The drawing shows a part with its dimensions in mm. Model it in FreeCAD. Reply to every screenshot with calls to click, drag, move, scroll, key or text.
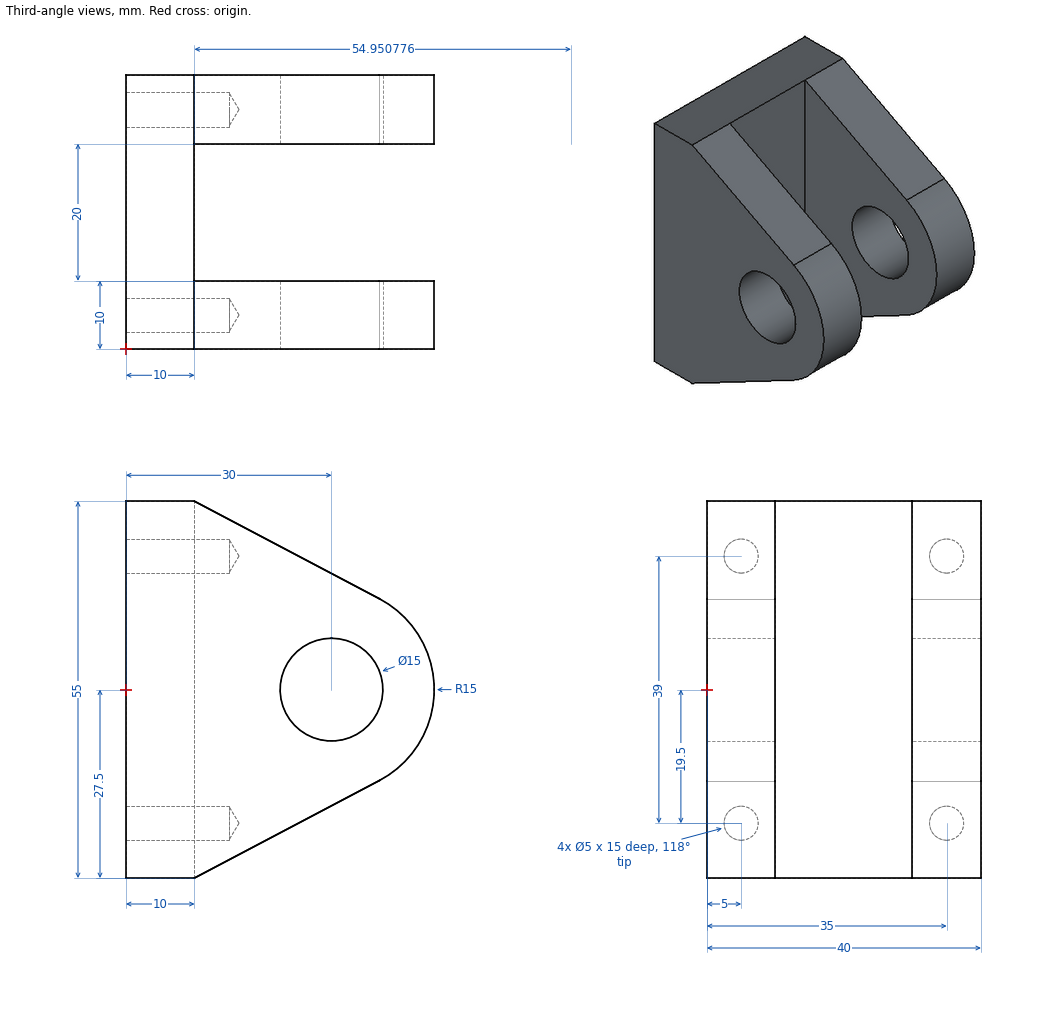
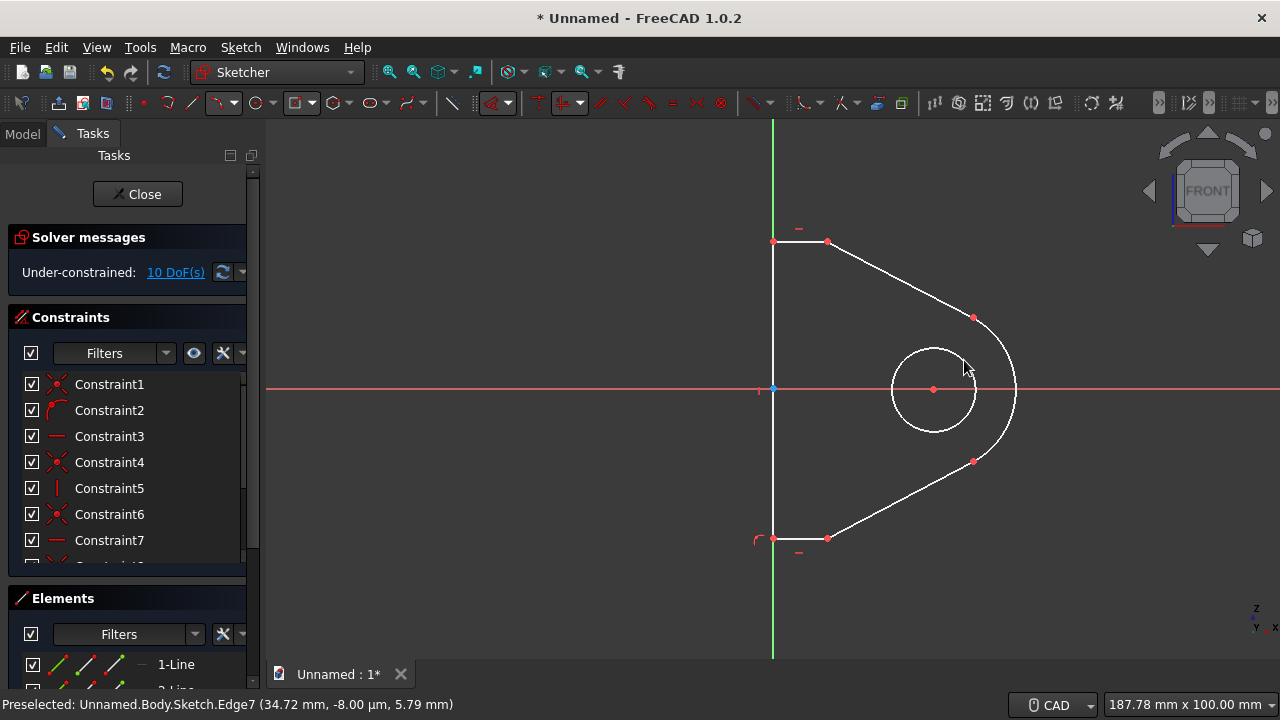
click(929, 485)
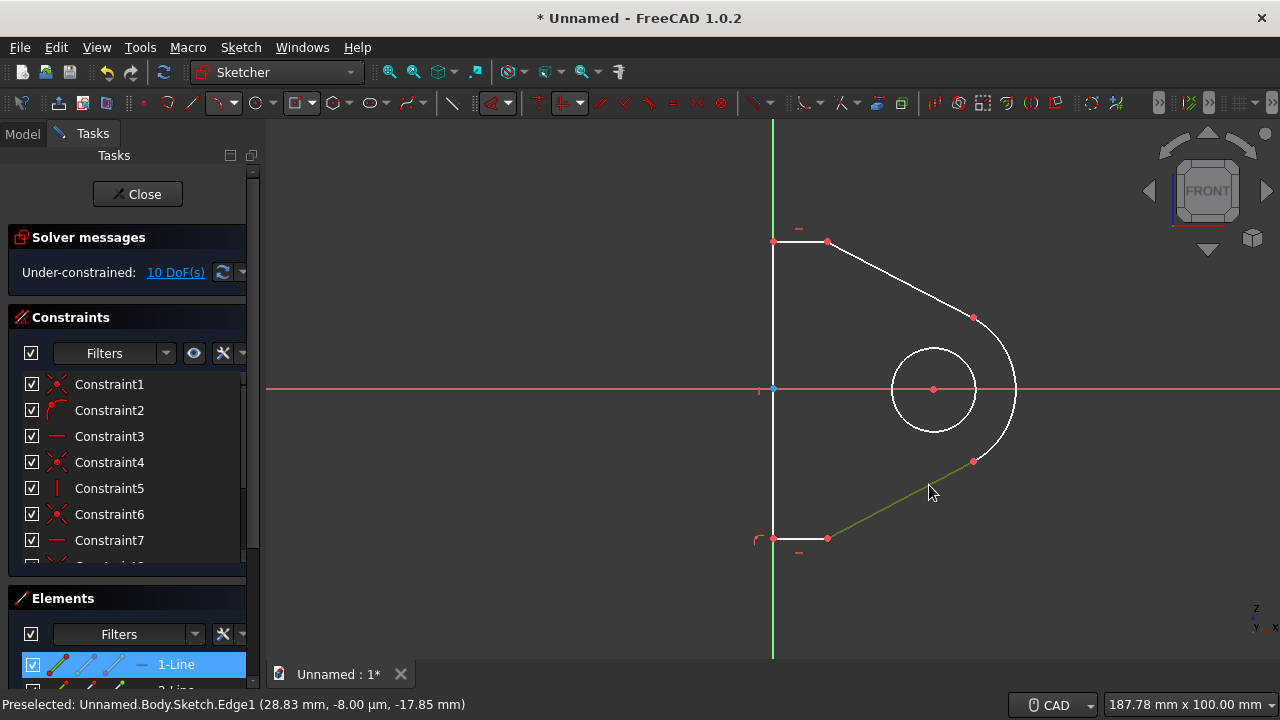
click(1008, 424)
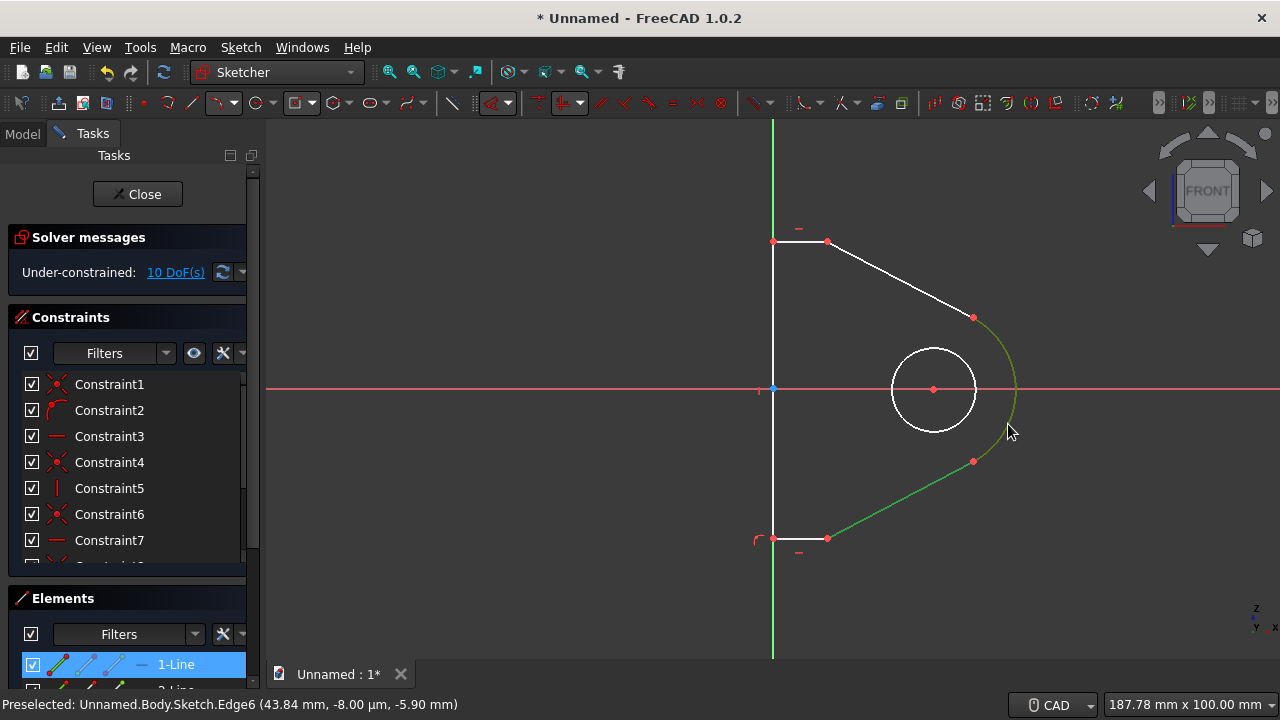
click(650, 104)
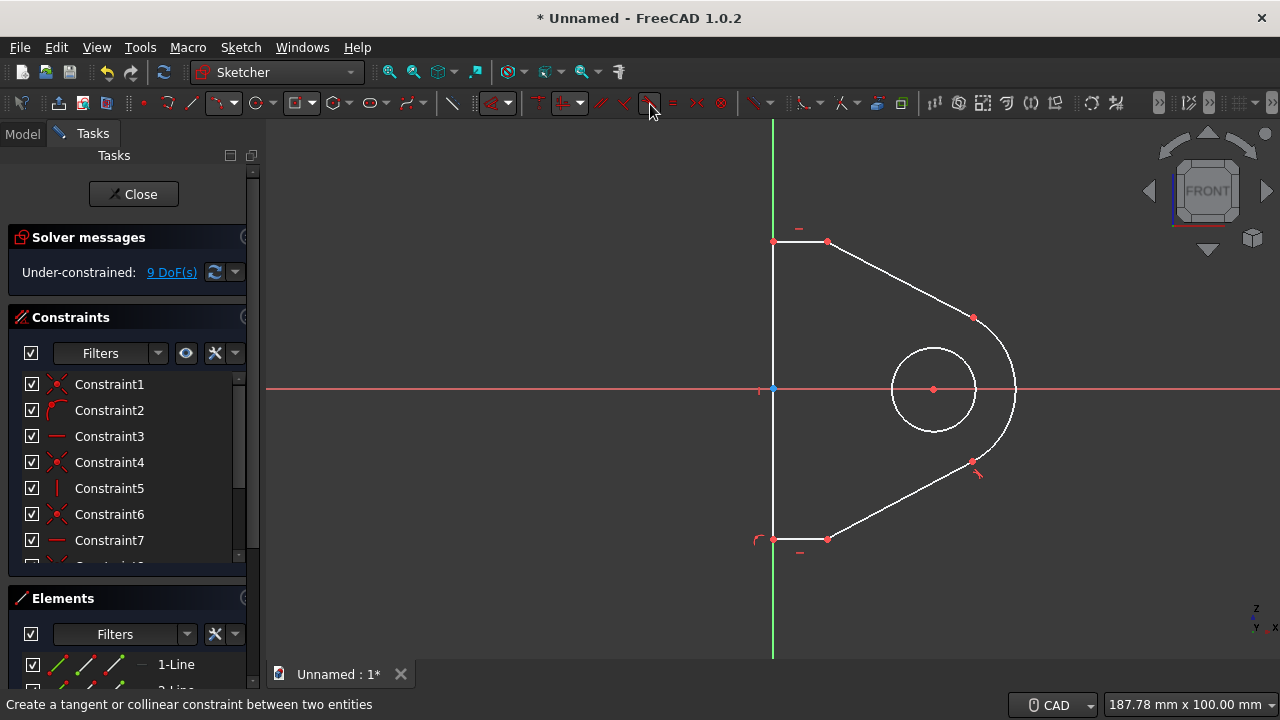
click(871, 265)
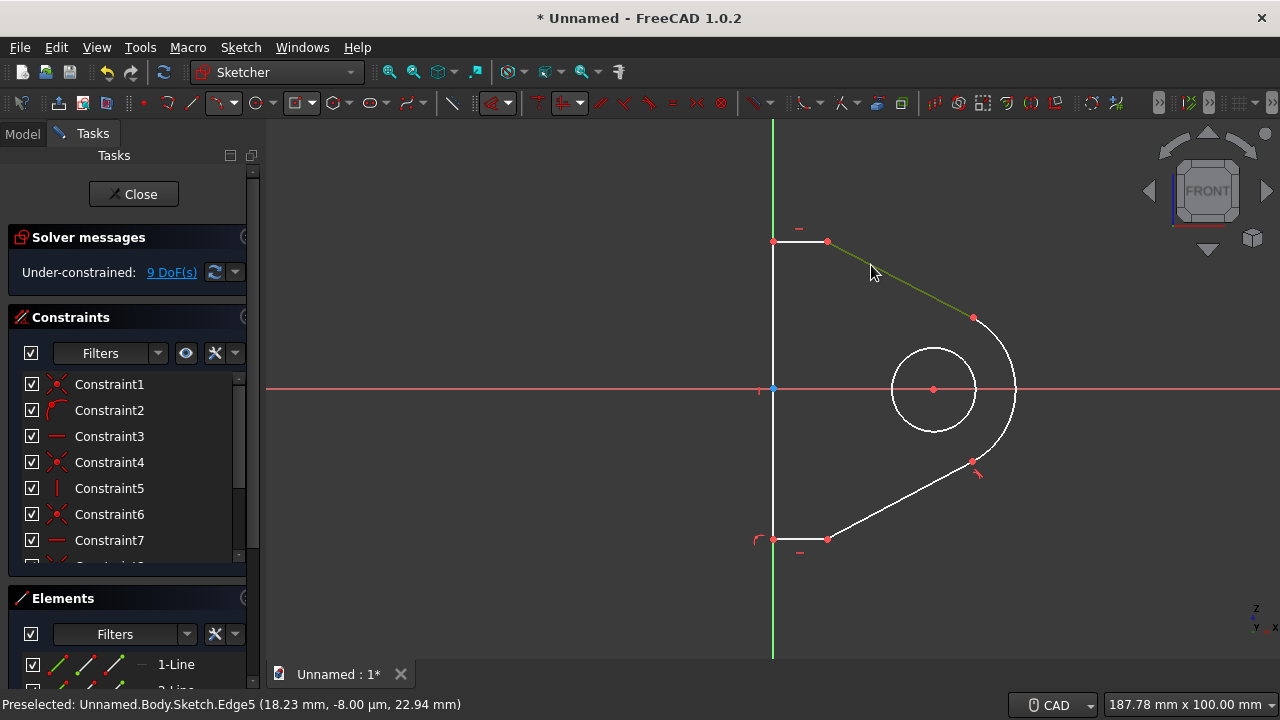
click(1008, 424)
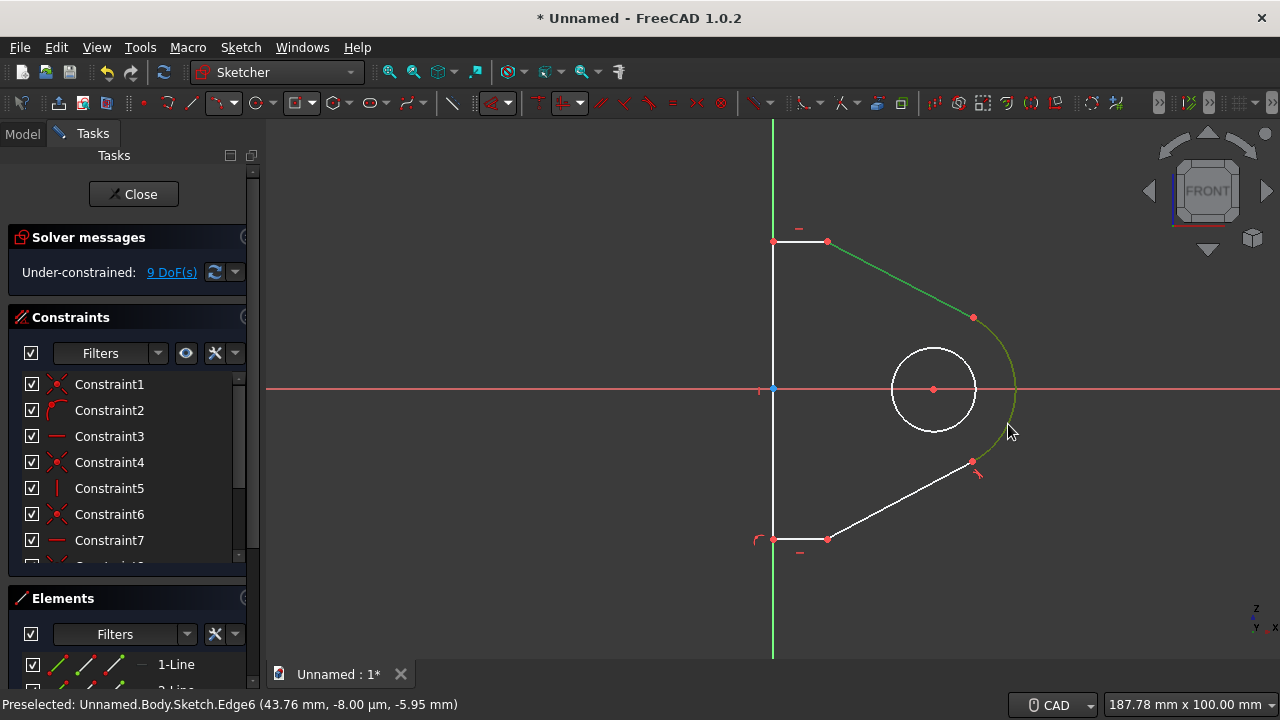
key(t)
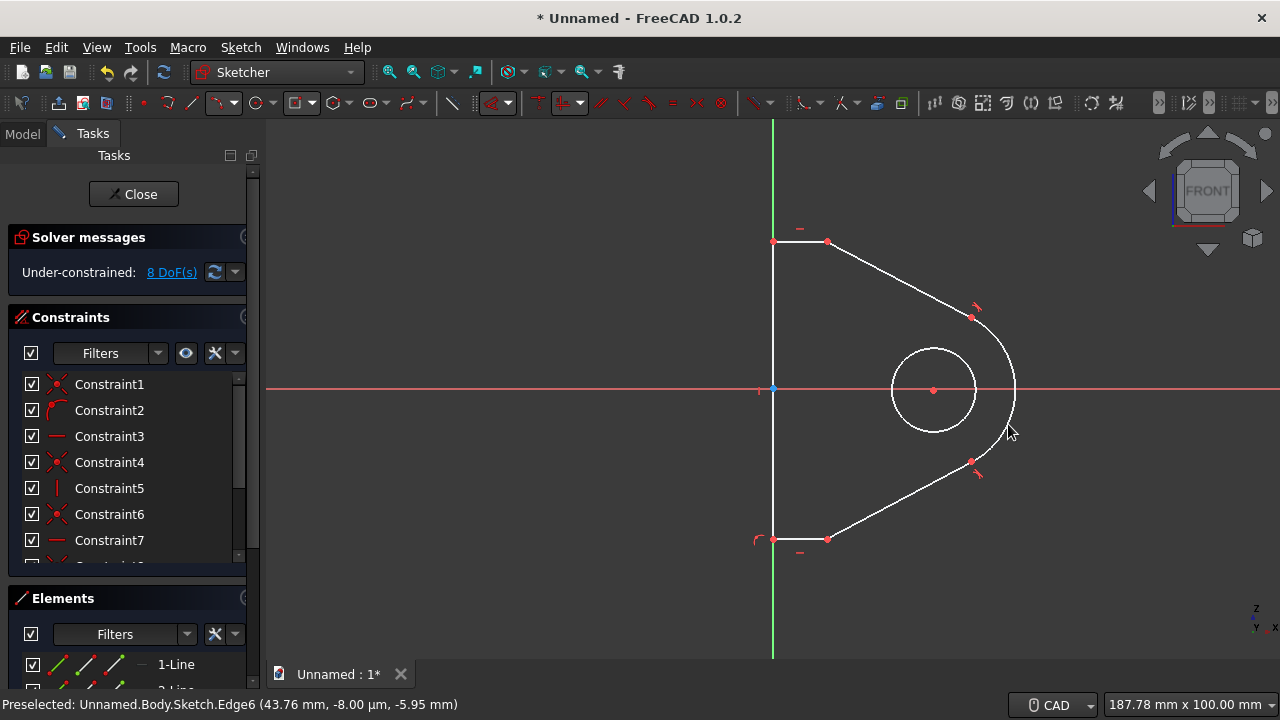
click(934, 390)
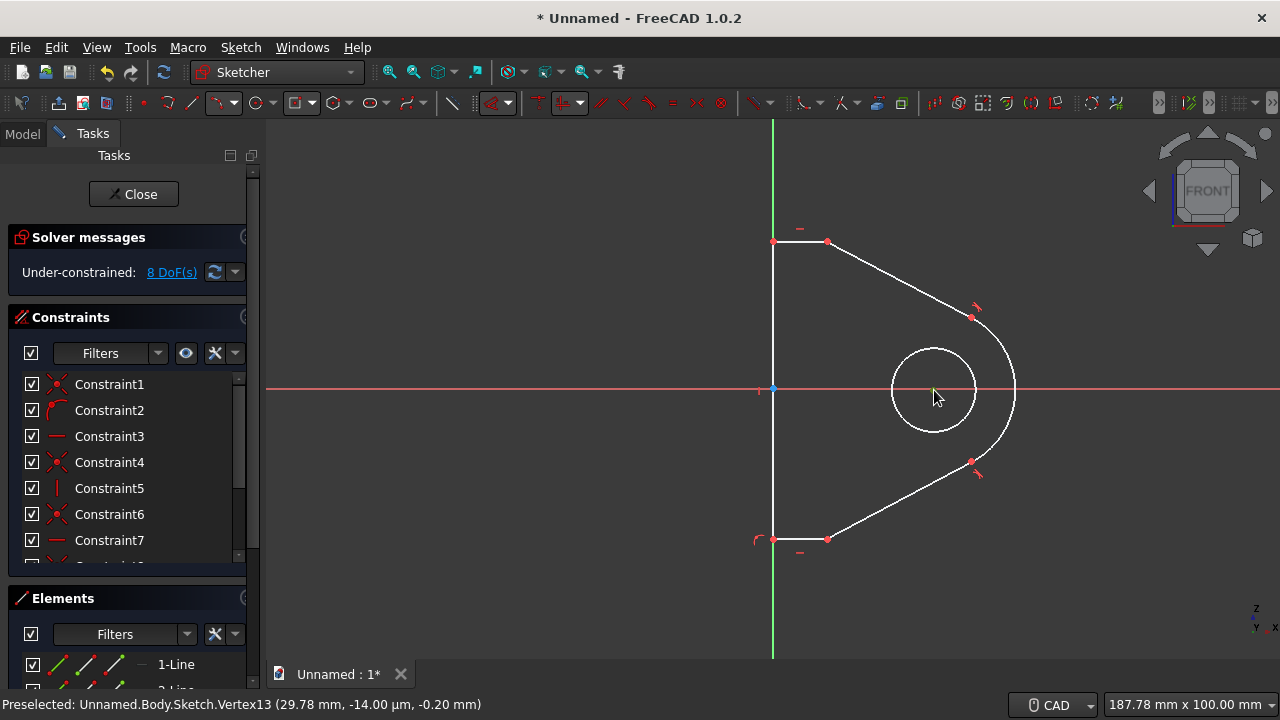
click(353, 389)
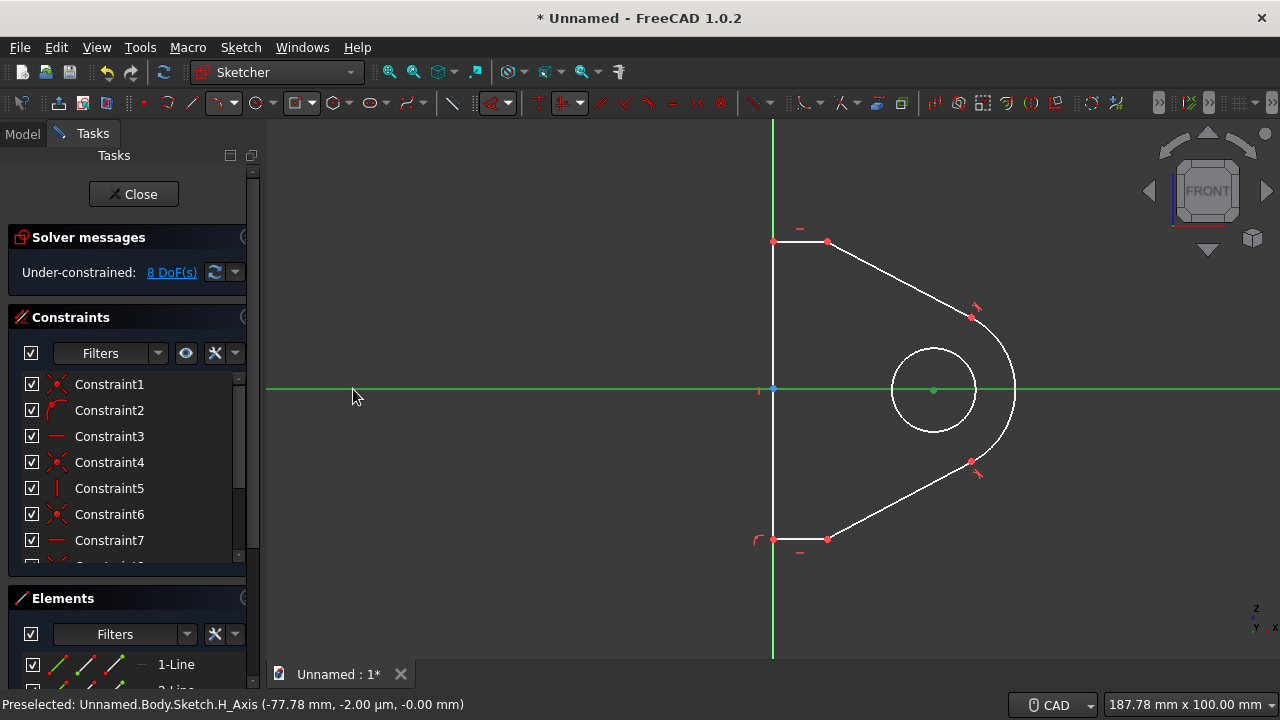
key(c)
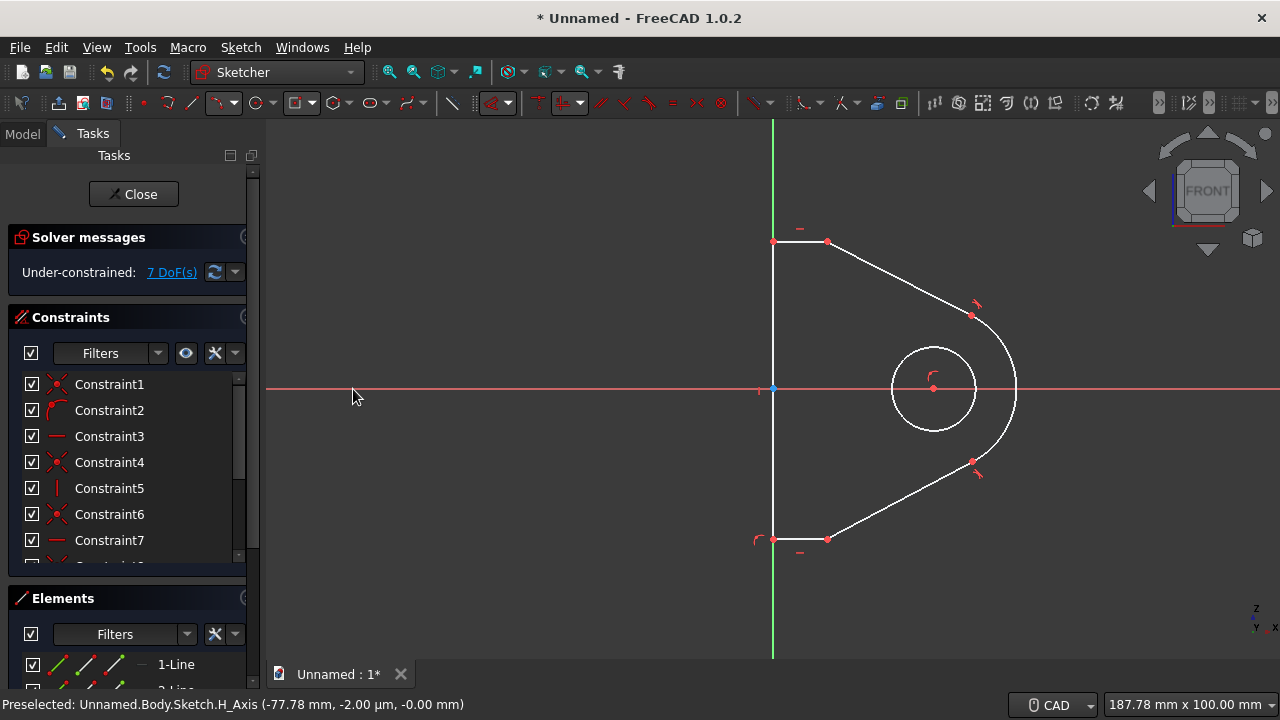
click(1009, 423)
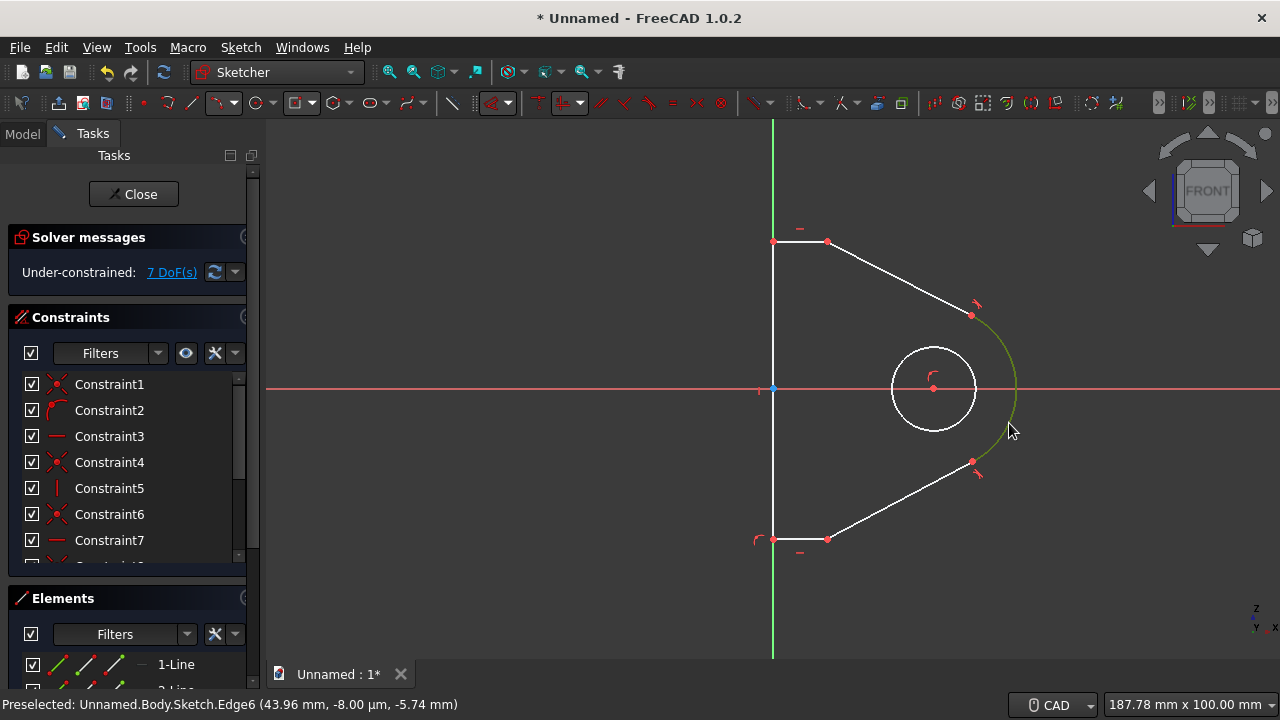
key(k)
key(r)